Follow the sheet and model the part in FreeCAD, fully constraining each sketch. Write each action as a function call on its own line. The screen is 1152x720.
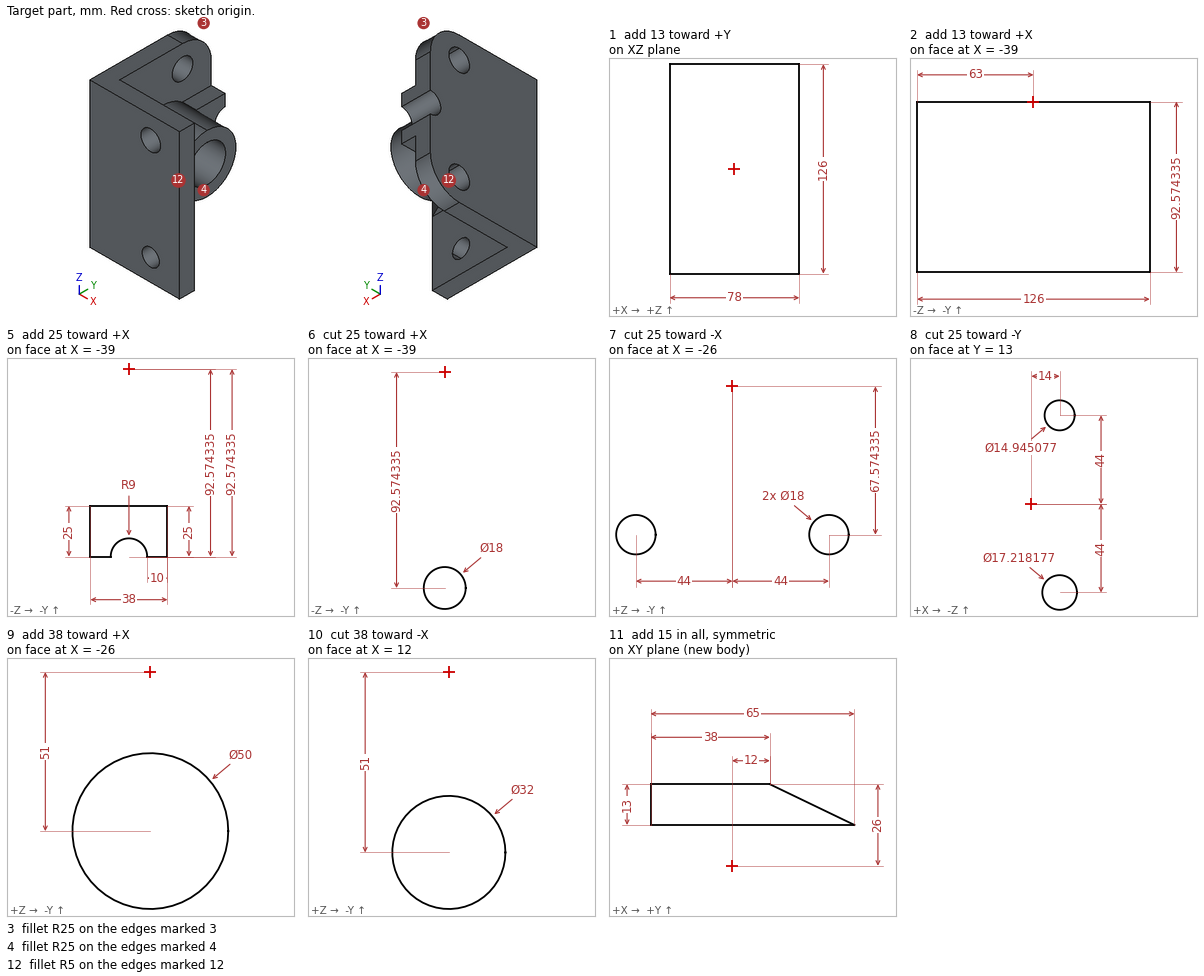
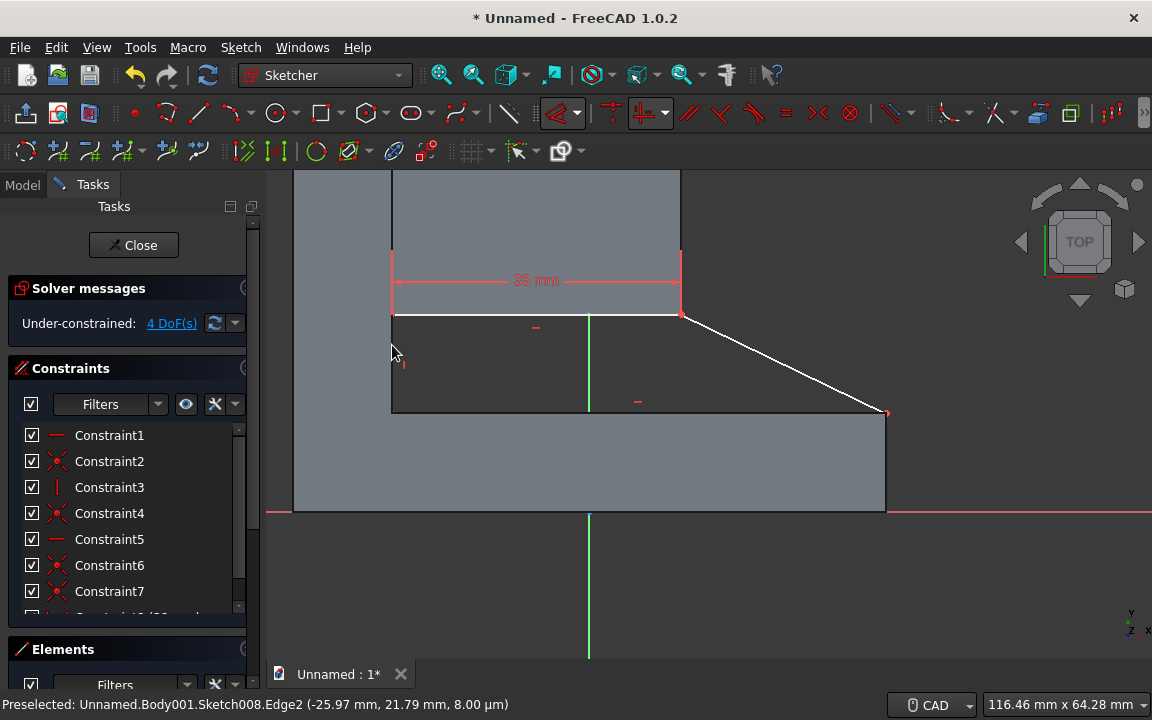
click(580, 114)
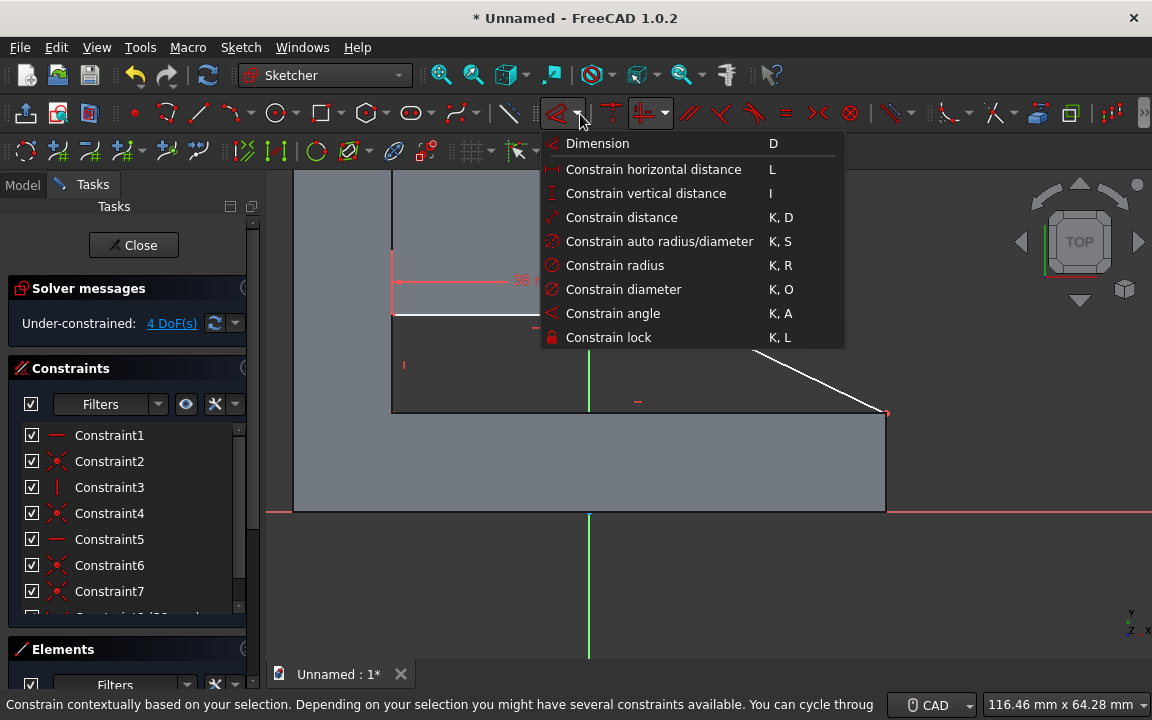
click(693, 193)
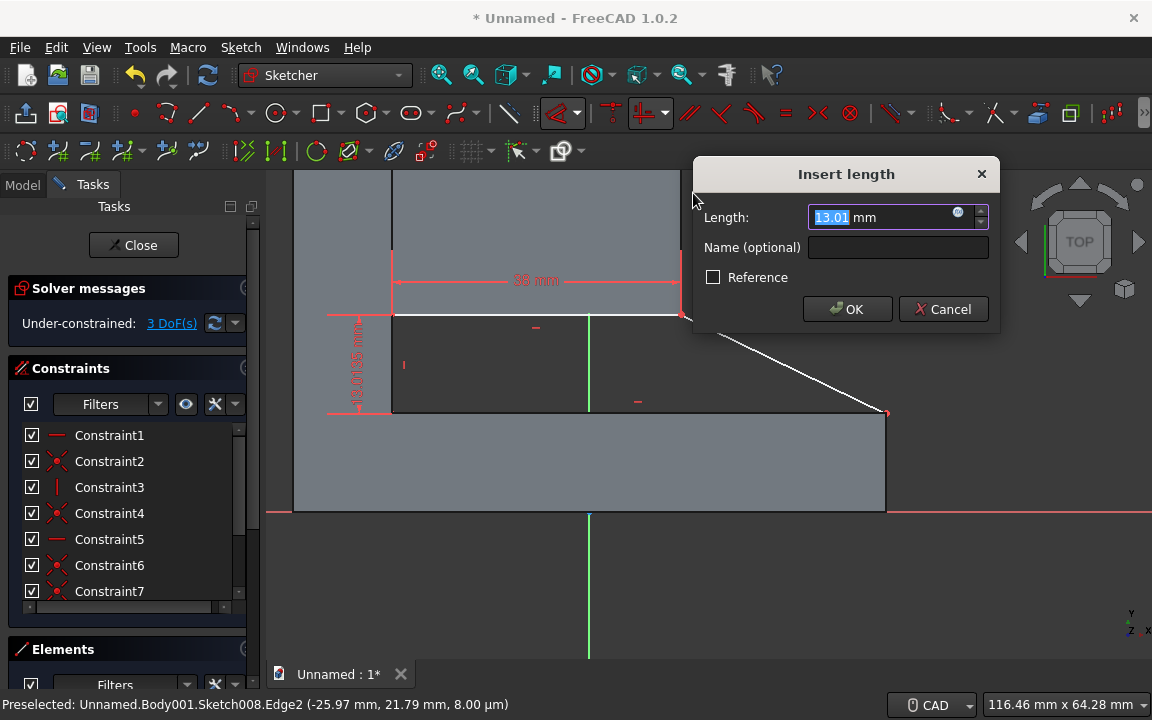
text(13)
key(Return)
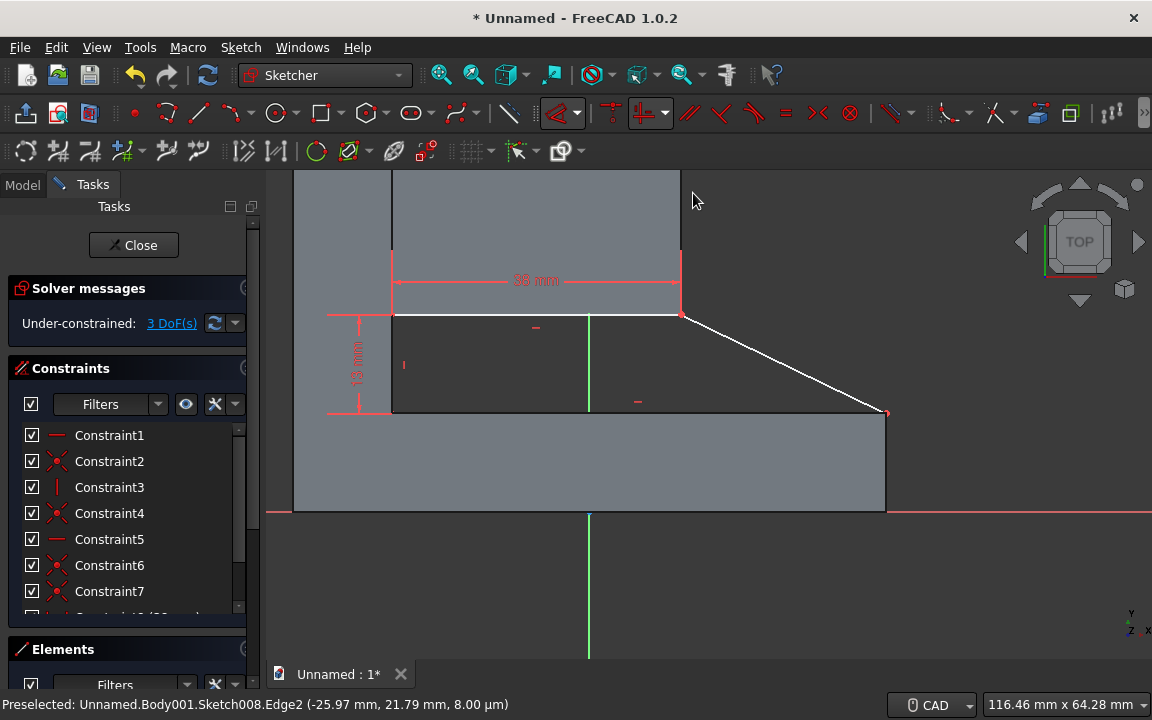
click(540, 414)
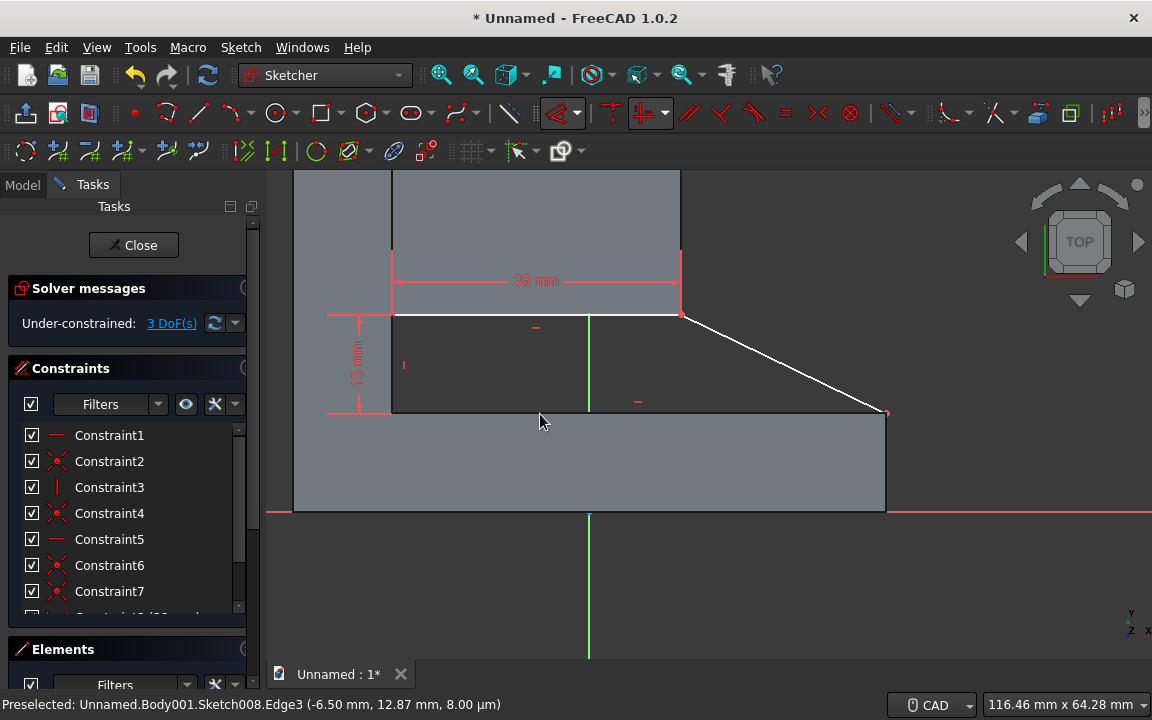
key(l)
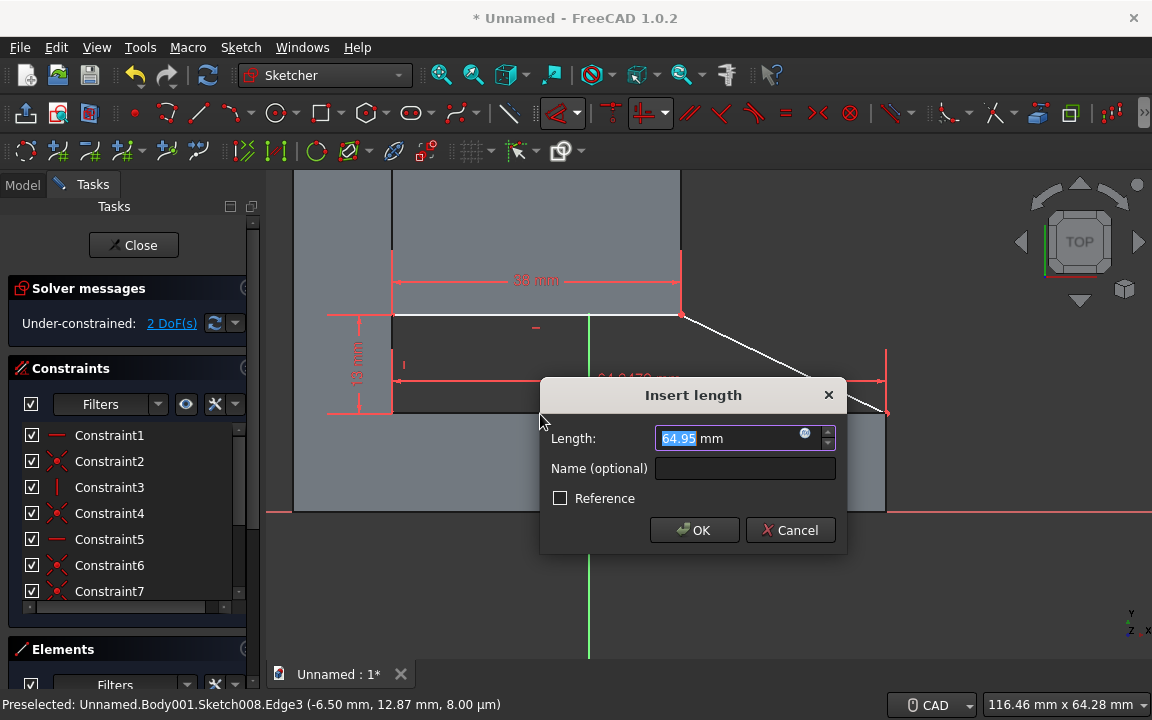
text(65)
key(Return)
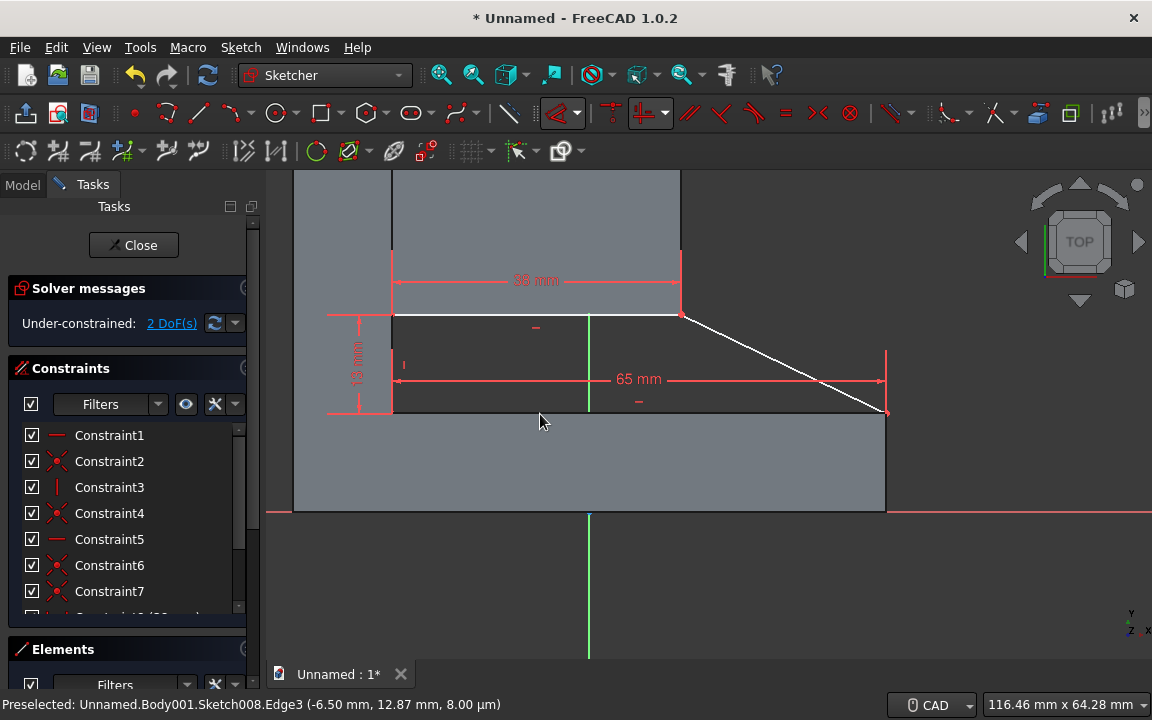
click(681, 315)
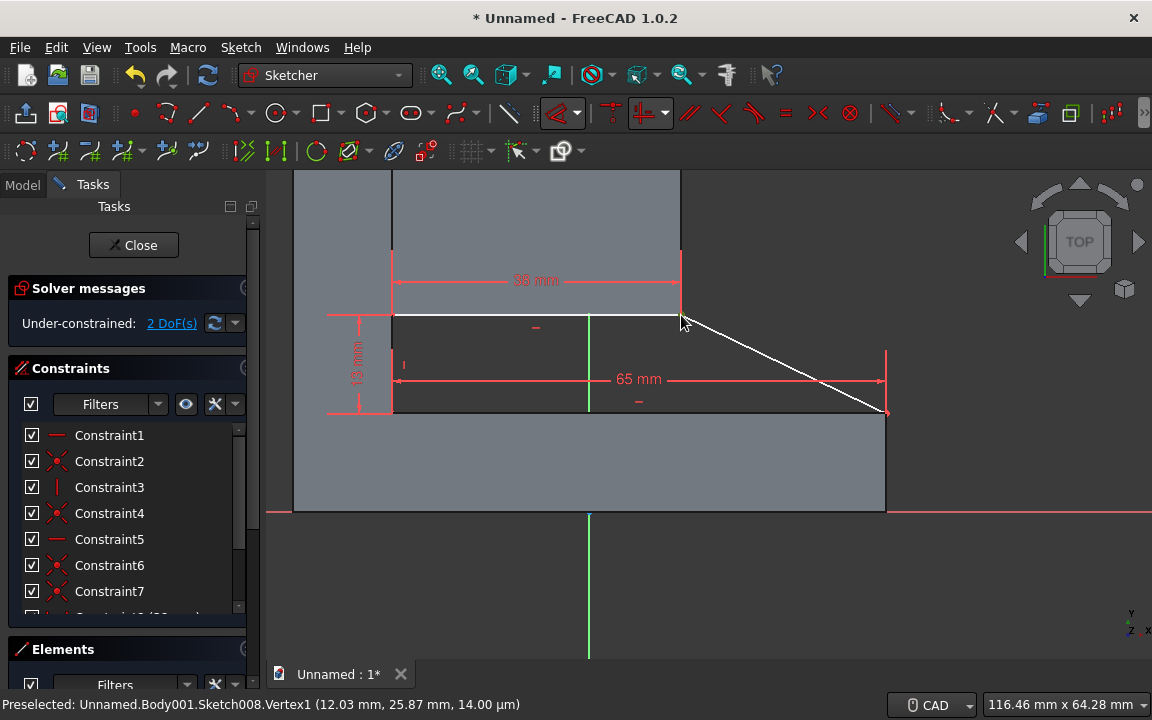
key(l)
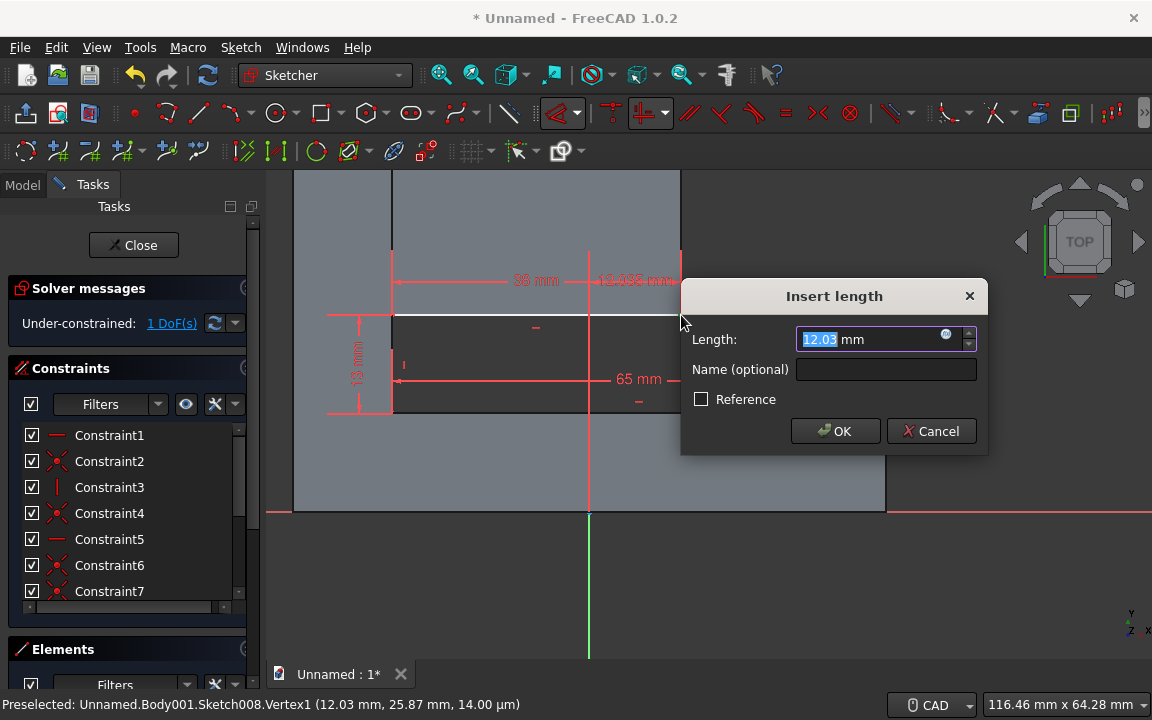
text(12)
key(Return)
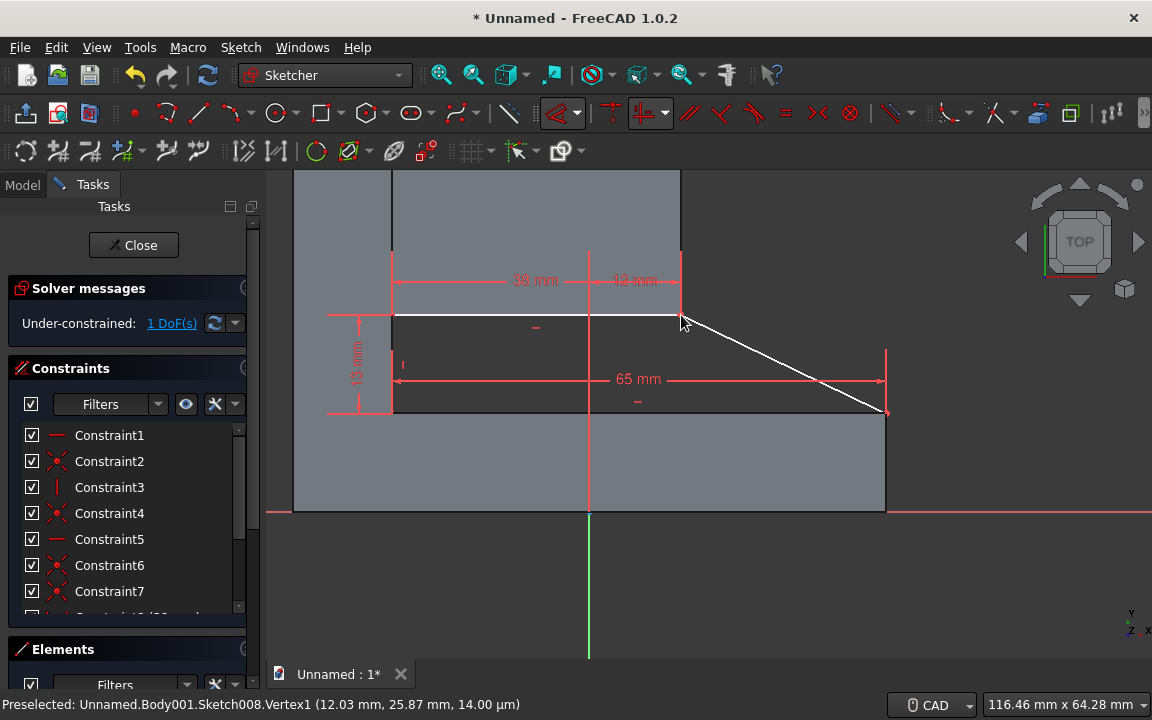
click(681, 315)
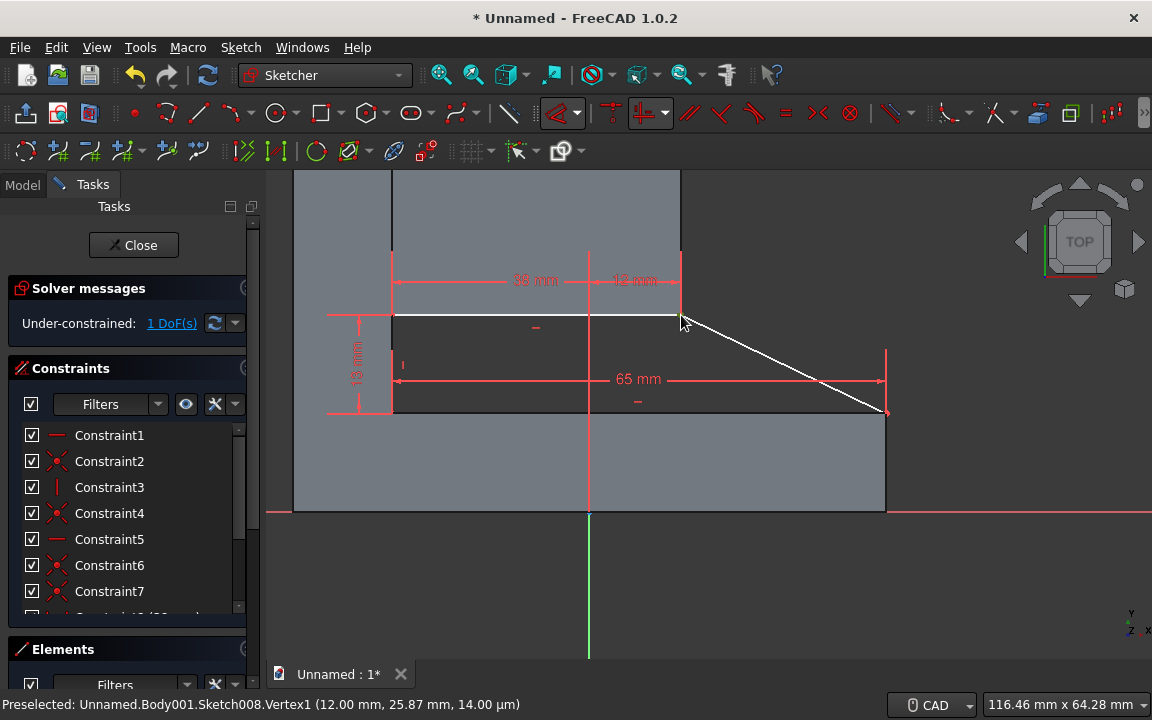
key(i)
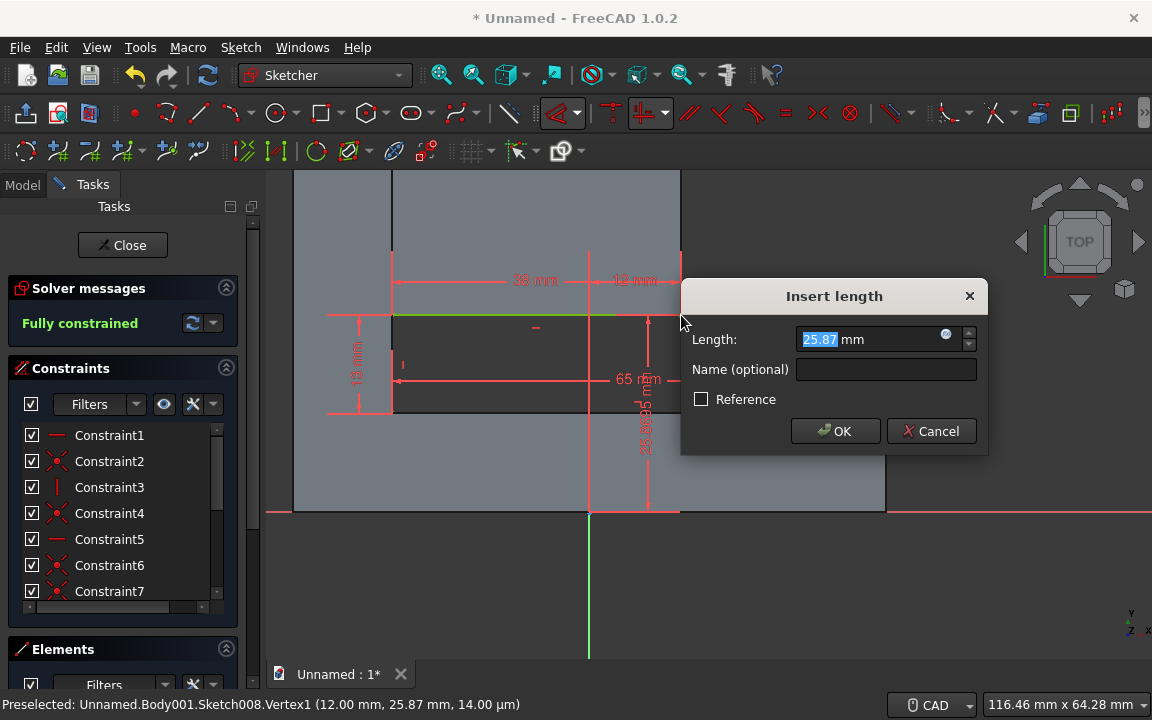
text(26)
key(Return)